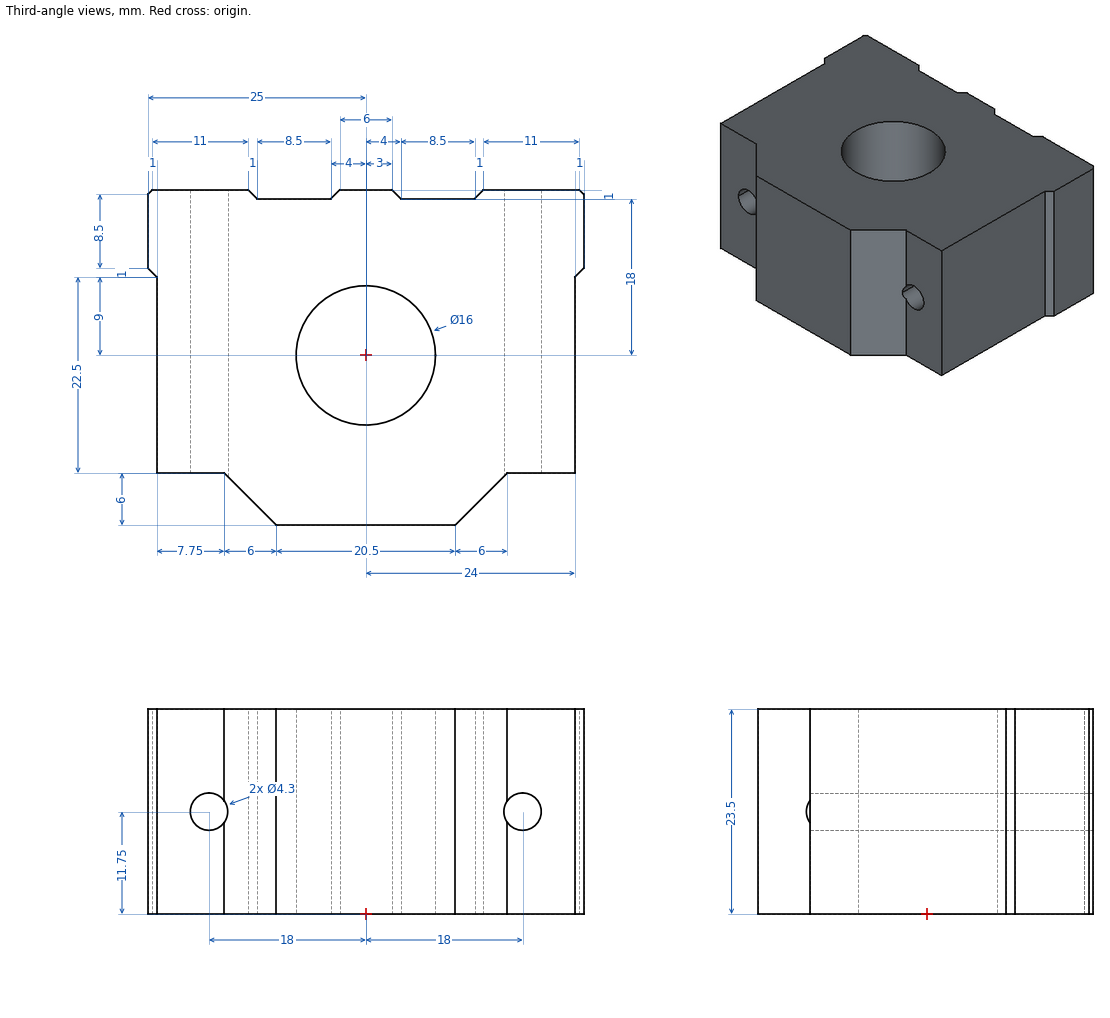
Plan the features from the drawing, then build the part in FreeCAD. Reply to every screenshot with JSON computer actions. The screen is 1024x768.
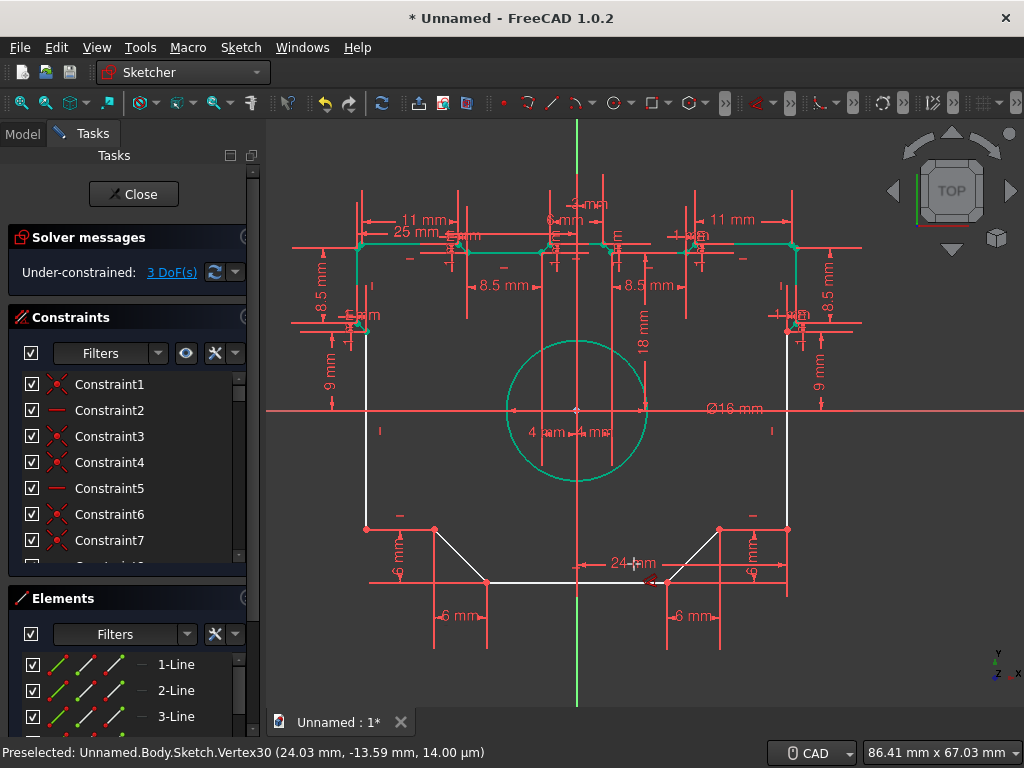
{"action": "left_click", "coordinate": [366, 391]}
{"action": "left_click", "coordinate": [332, 431]}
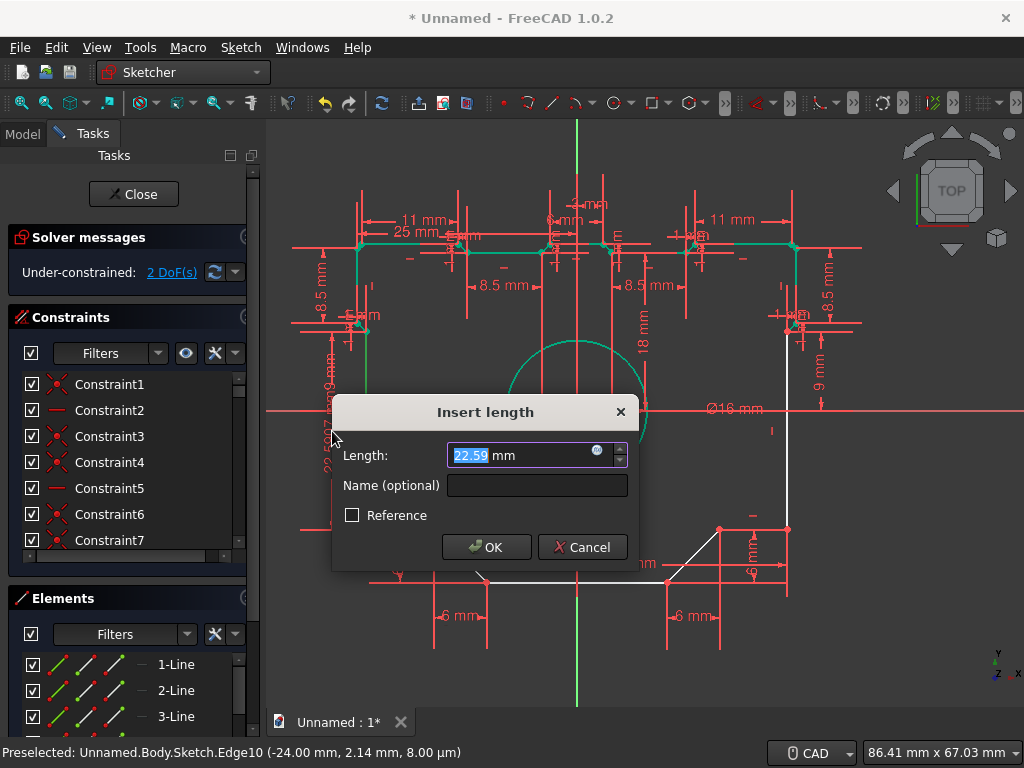
{"action": "type", "text": "22.5"}
{"action": "key", "text": "Return"}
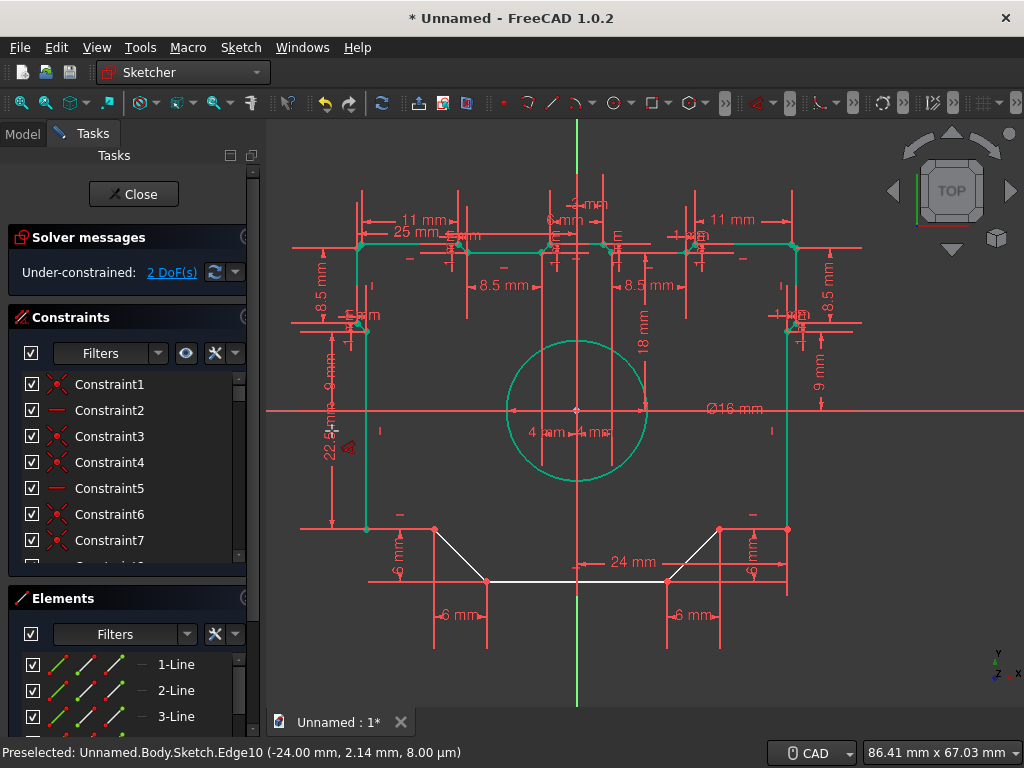
{"action": "left_click", "coordinate": [387, 529]}
{"action": "left_click", "coordinate": [400, 495]}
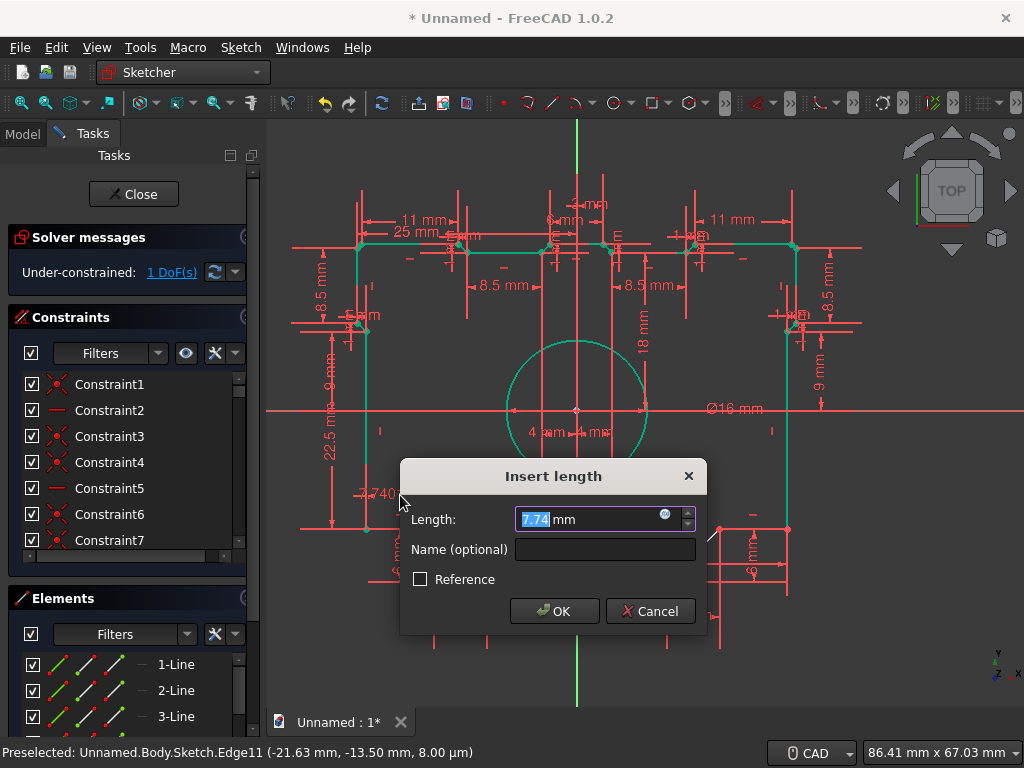
{"action": "type", "text": "7.75"}
{"action": "key", "text": "Return"}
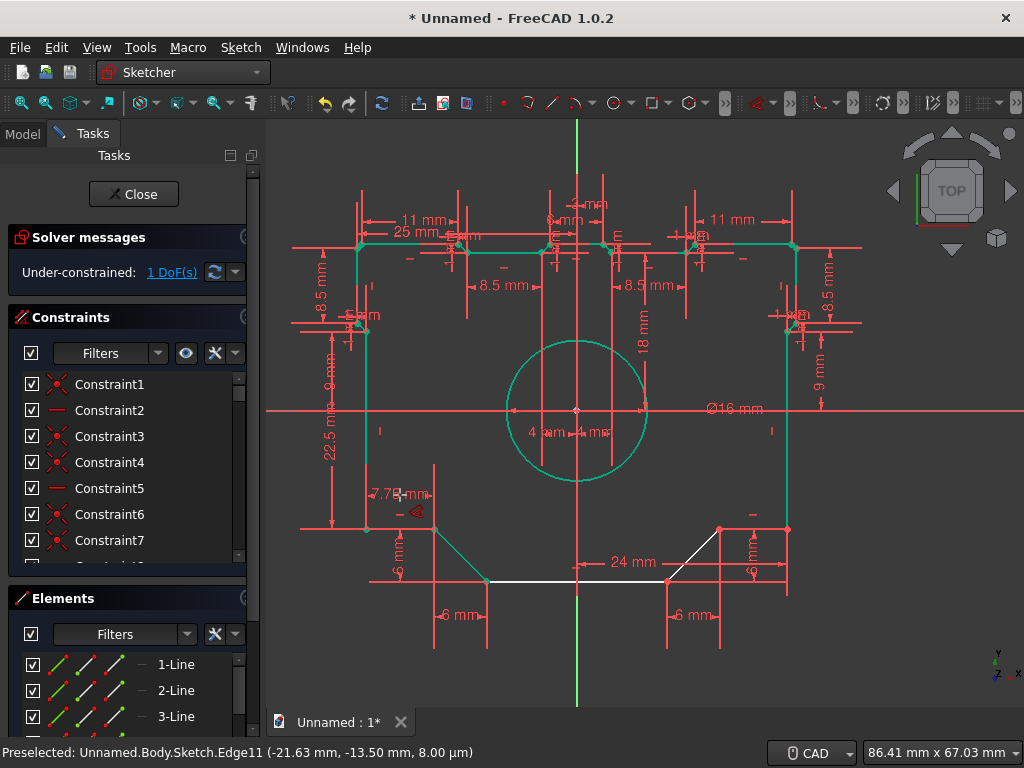
{"action": "left_click", "coordinate": [541, 582]}
{"action": "left_click", "coordinate": [536, 616]}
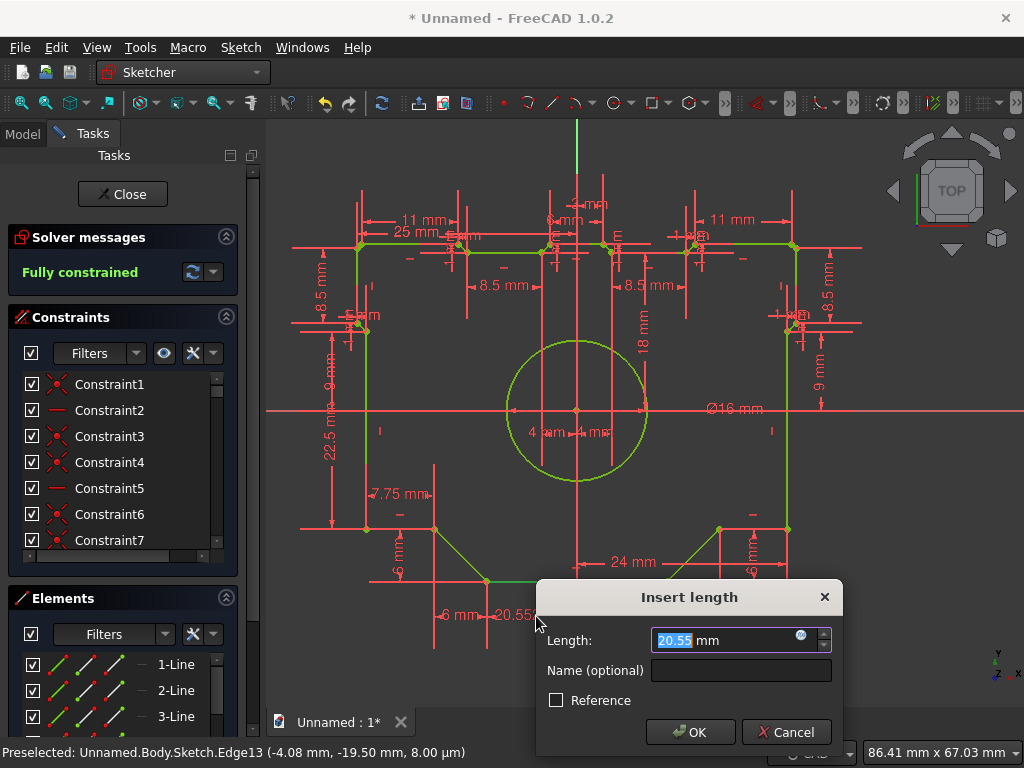
{"action": "type", "text": "20.5"}
{"action": "key", "text": "Return"}
{"action": "key", "text": "Escape"}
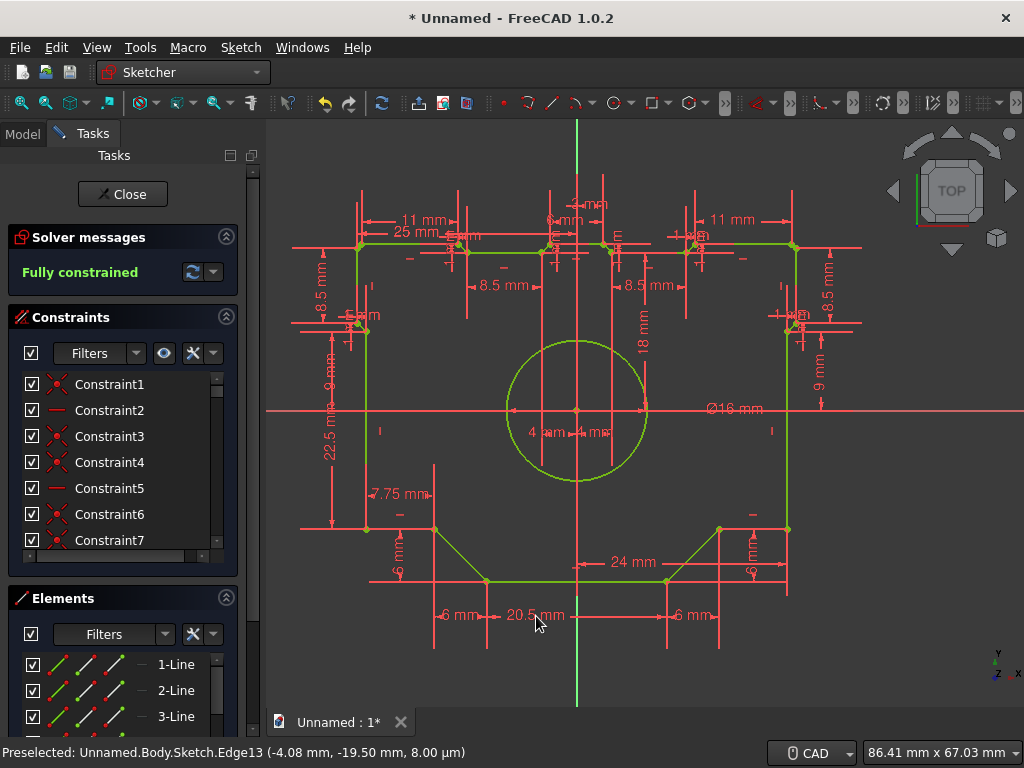
{"action": "left_click", "coordinate": [123, 194]}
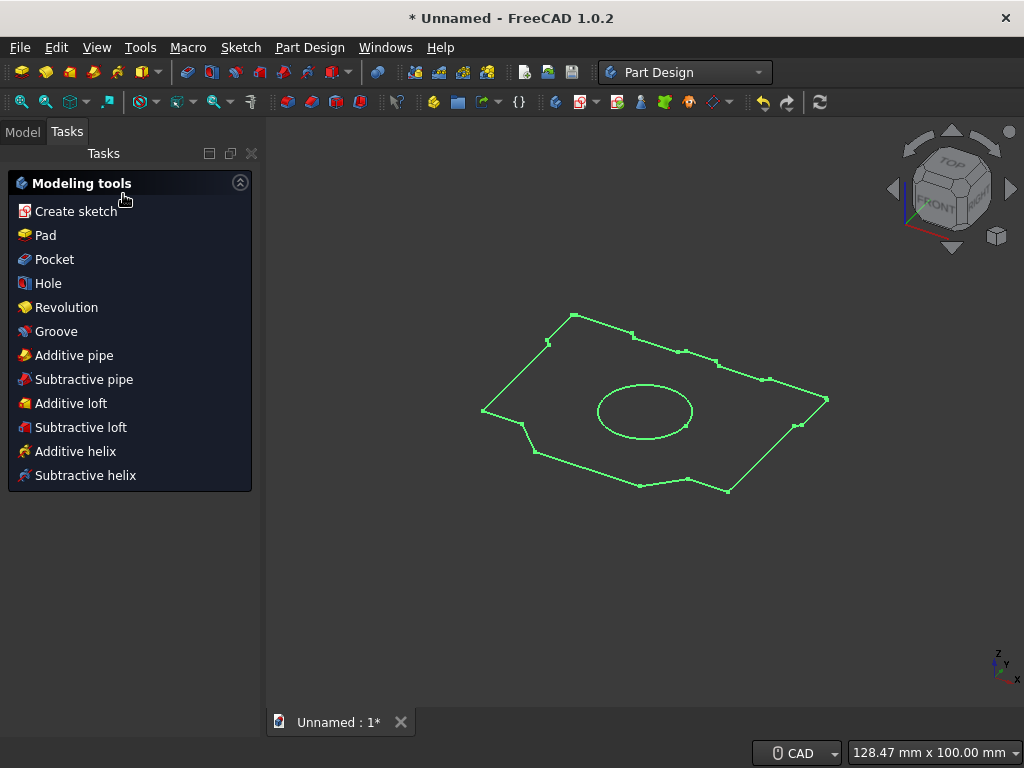
{"action": "left_click", "coordinate": [22, 72]}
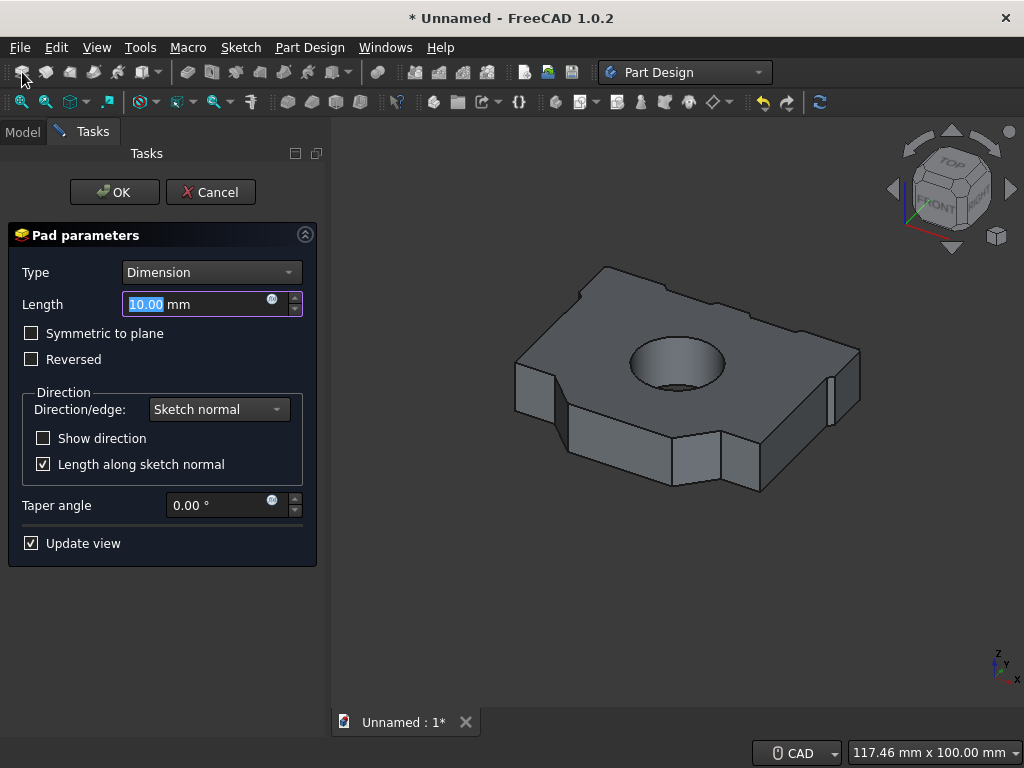
{"action": "type", "text": "23.5"}
{"action": "key", "text": "Tab"}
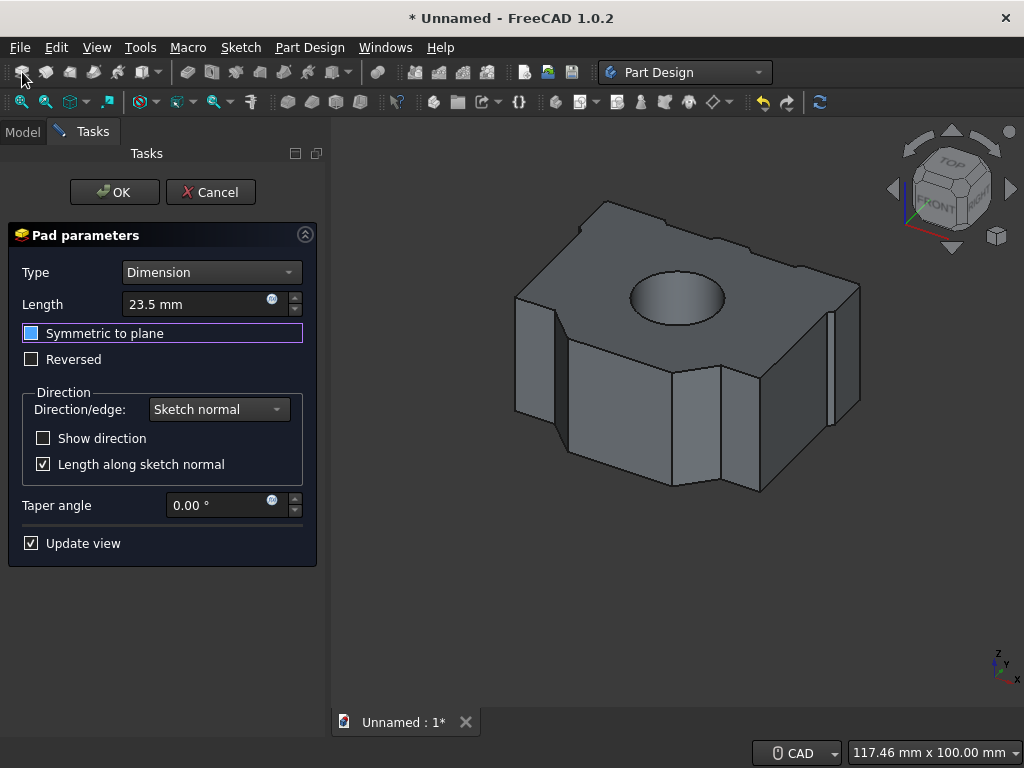
{"action": "left_click", "coordinate": [115, 192]}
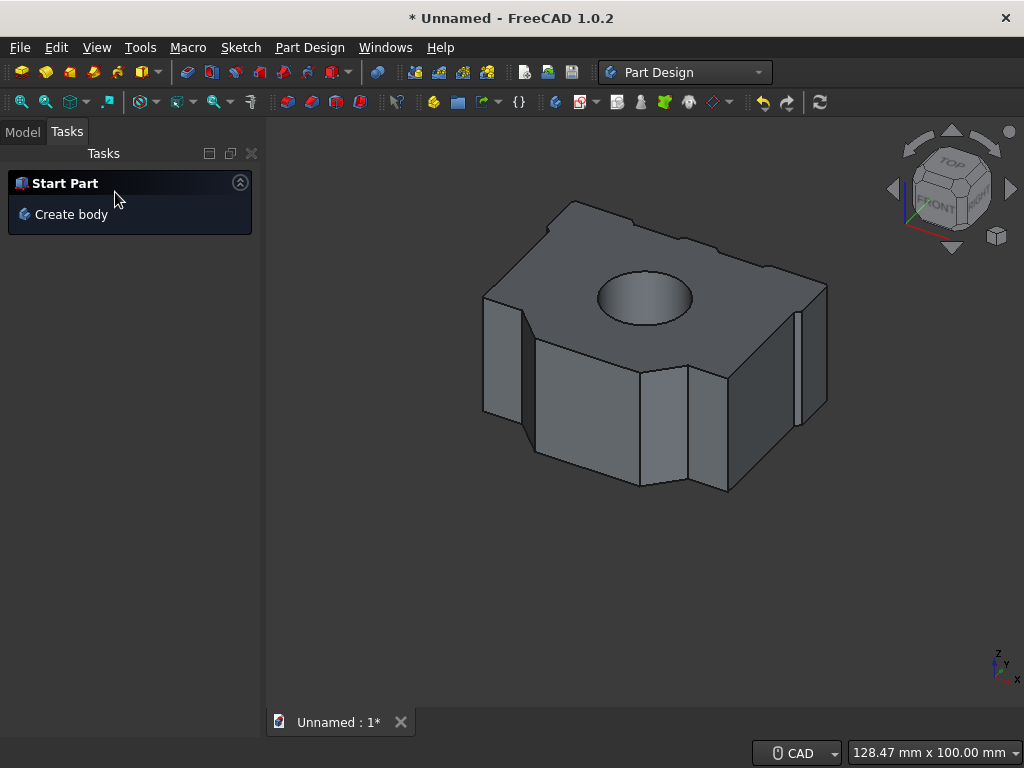
{"action": "key", "text": "4"}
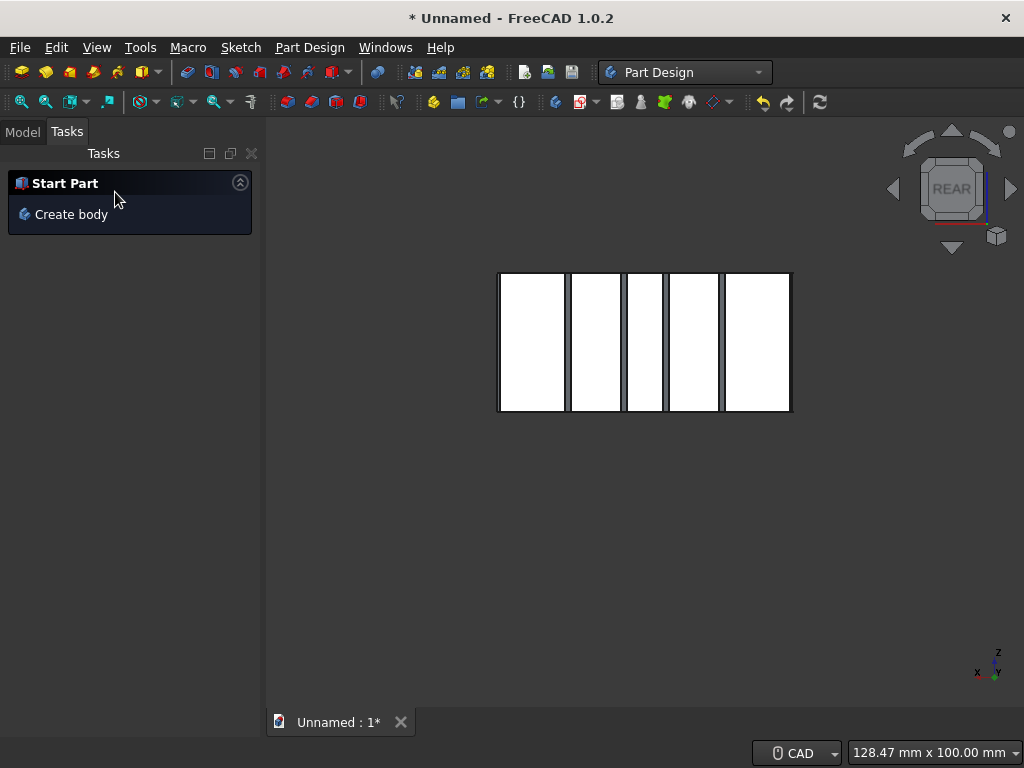
{"action": "left_click", "coordinate": [22, 102]}